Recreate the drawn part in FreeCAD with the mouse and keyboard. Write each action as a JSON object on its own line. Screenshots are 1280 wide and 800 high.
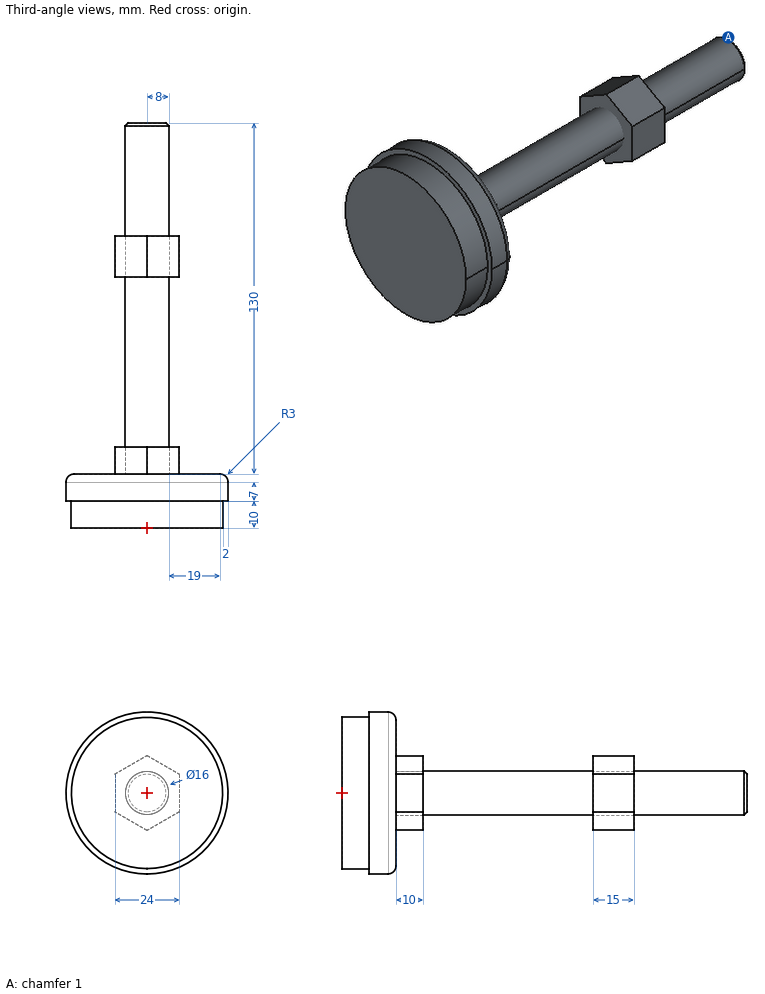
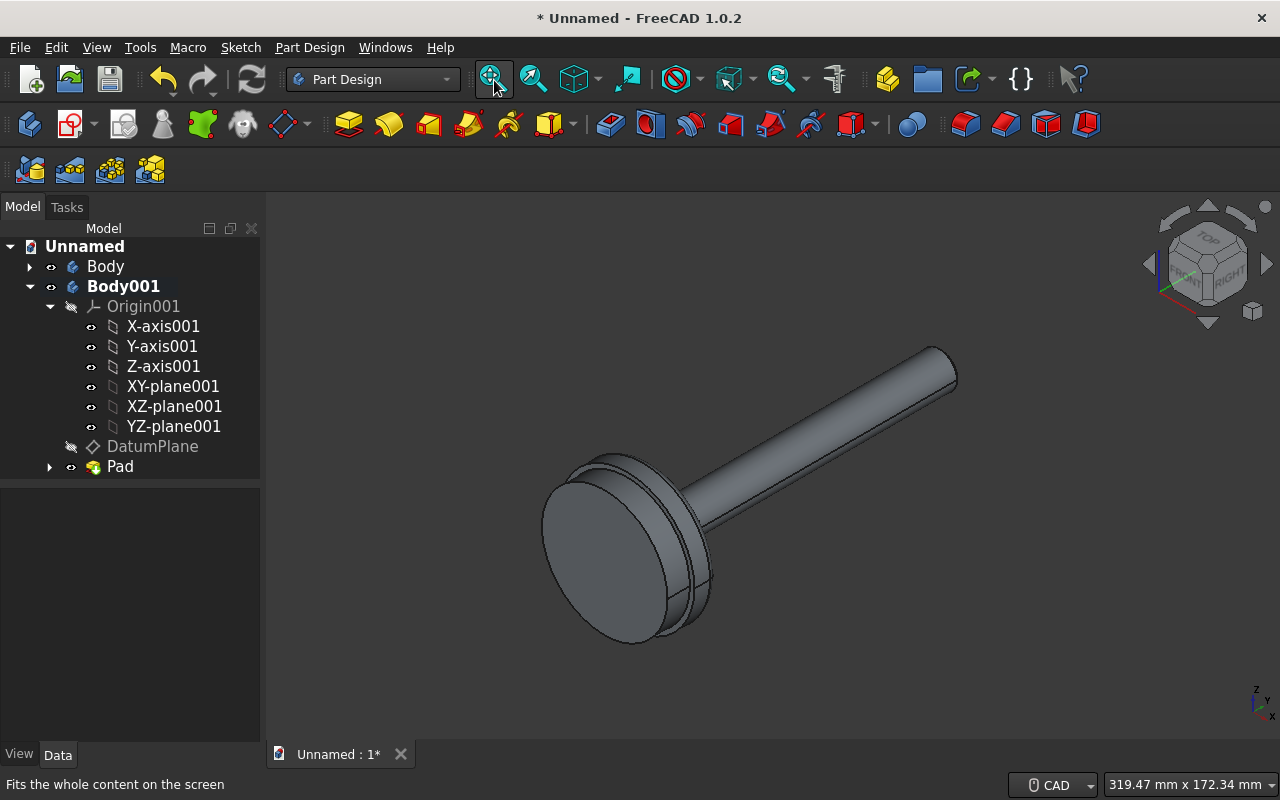
{"action": "left_click", "coordinate": [30, 124]}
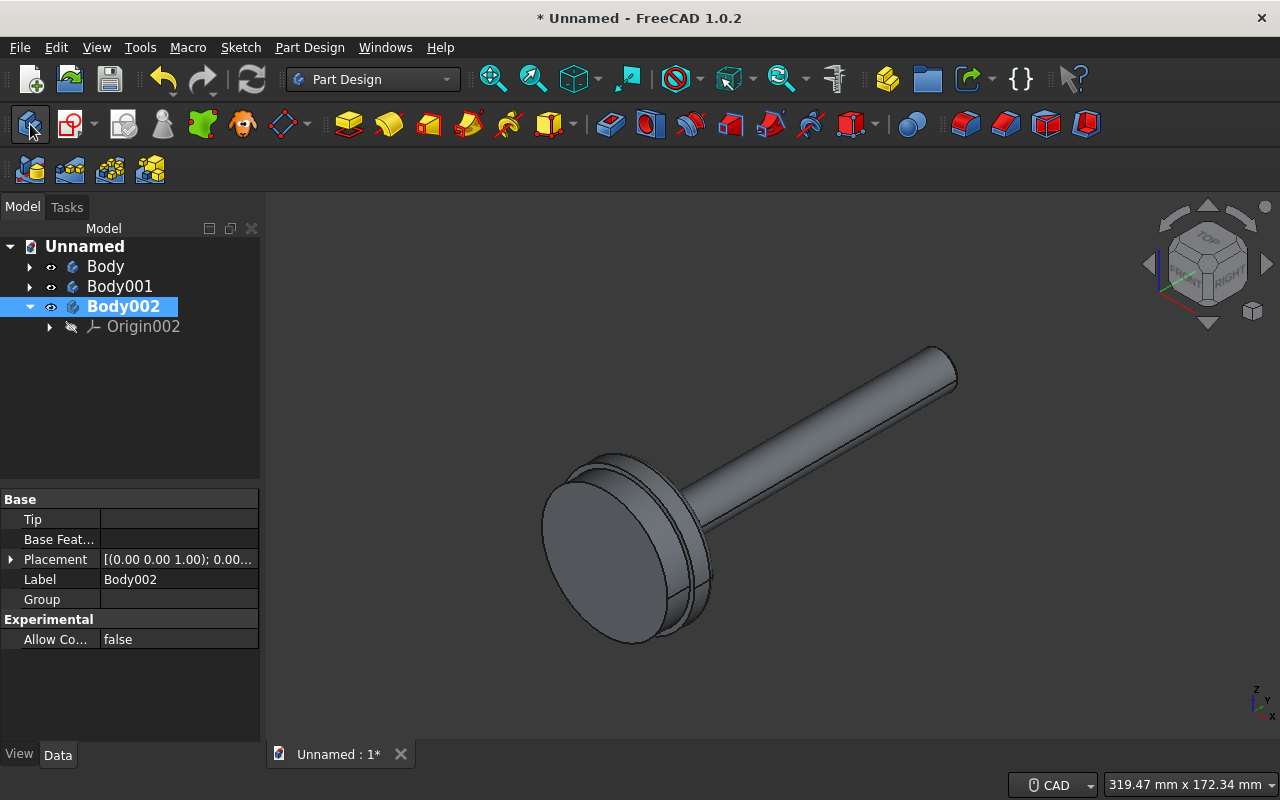
{"action": "left_click", "coordinate": [50, 327]}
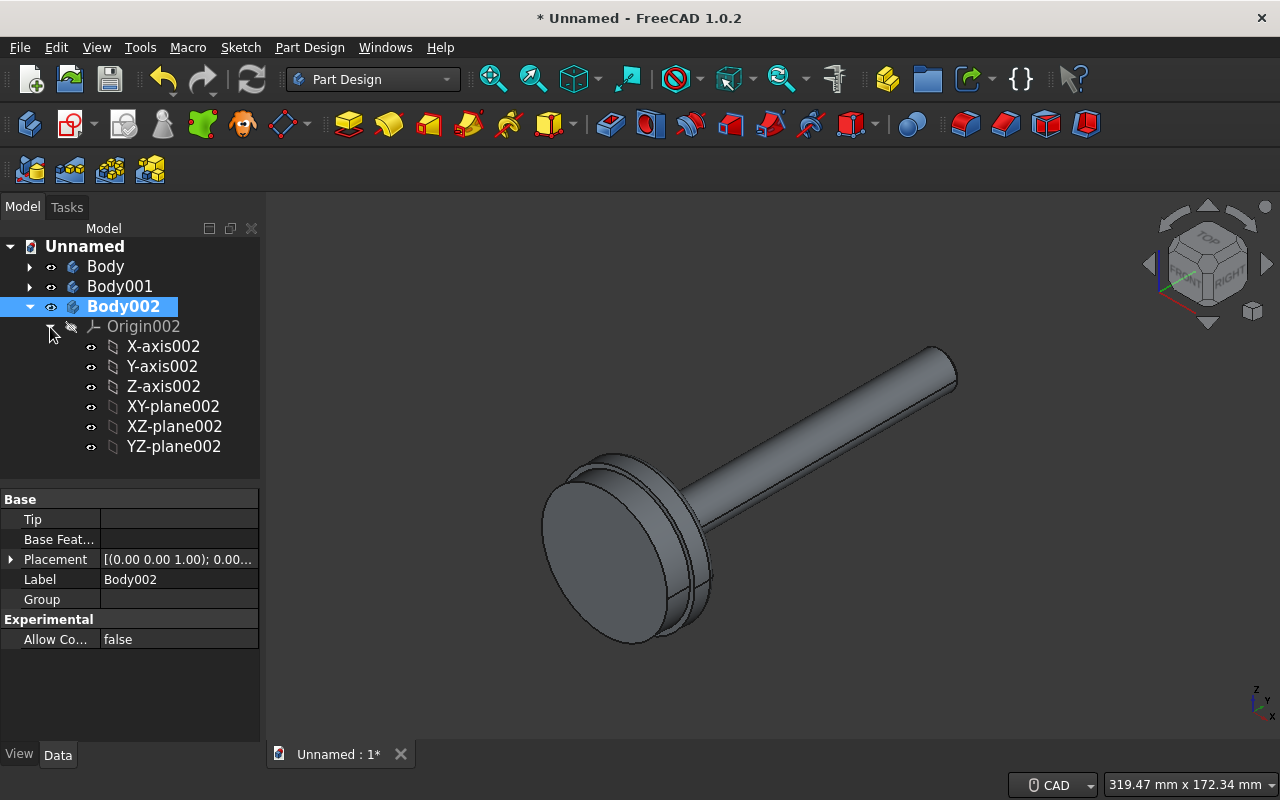
{"action": "left_click", "coordinate": [136, 427]}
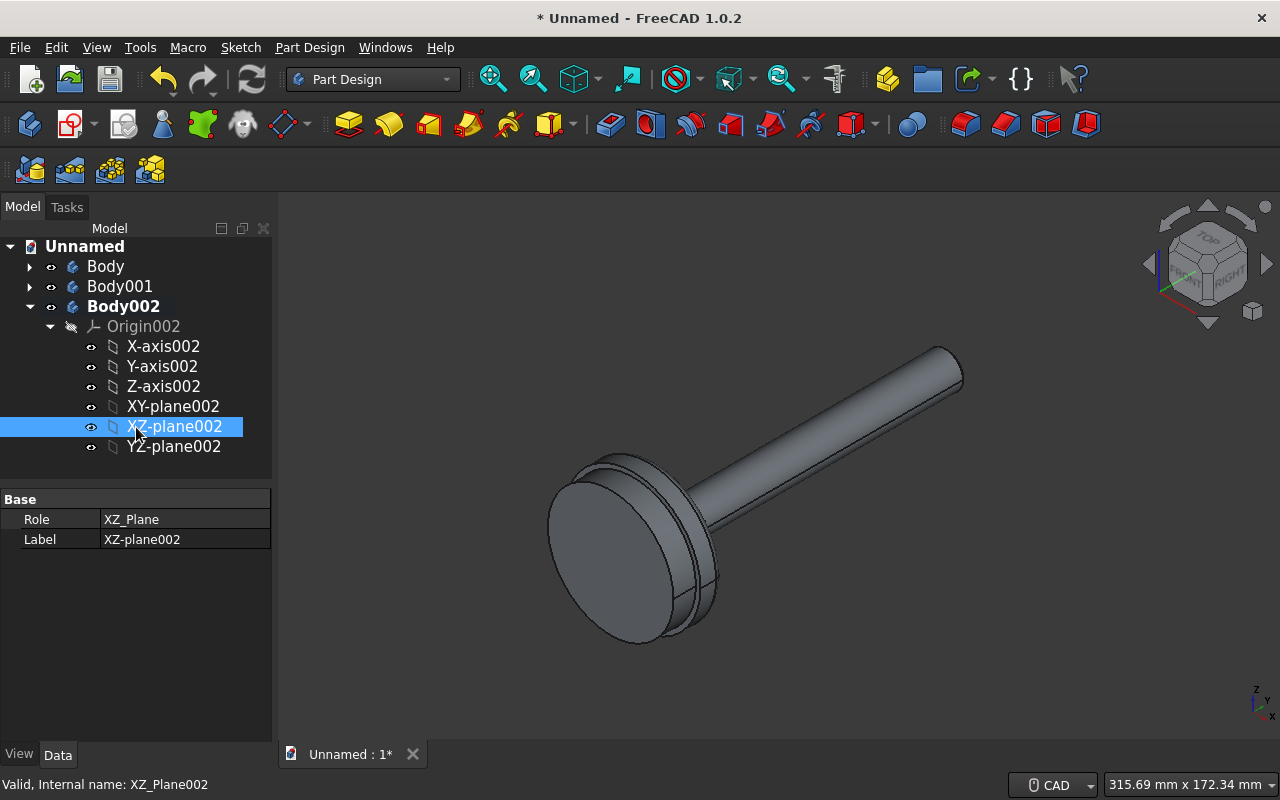
{"action": "left_click", "coordinate": [284, 124]}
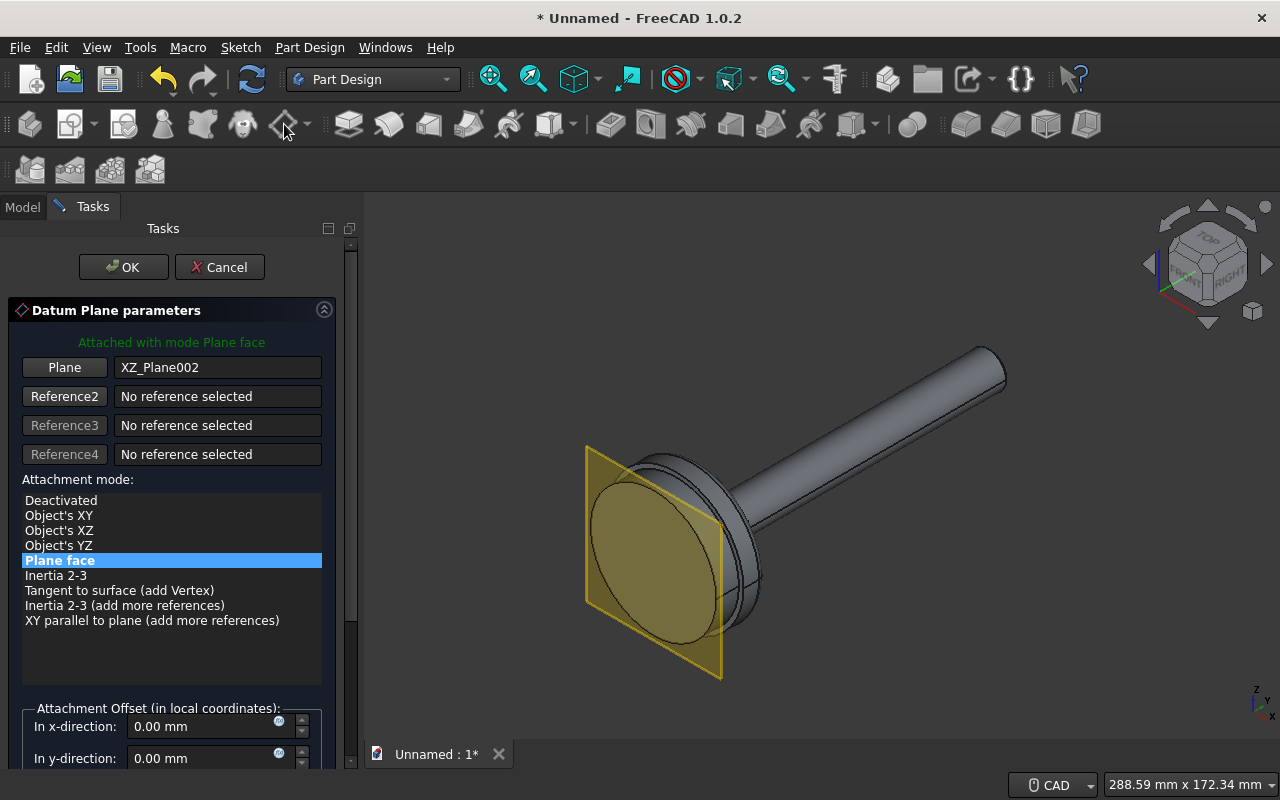
{"action": "scroll", "coordinate": [351, 503], "scroll_direction": "down", "scroll_amount": 2}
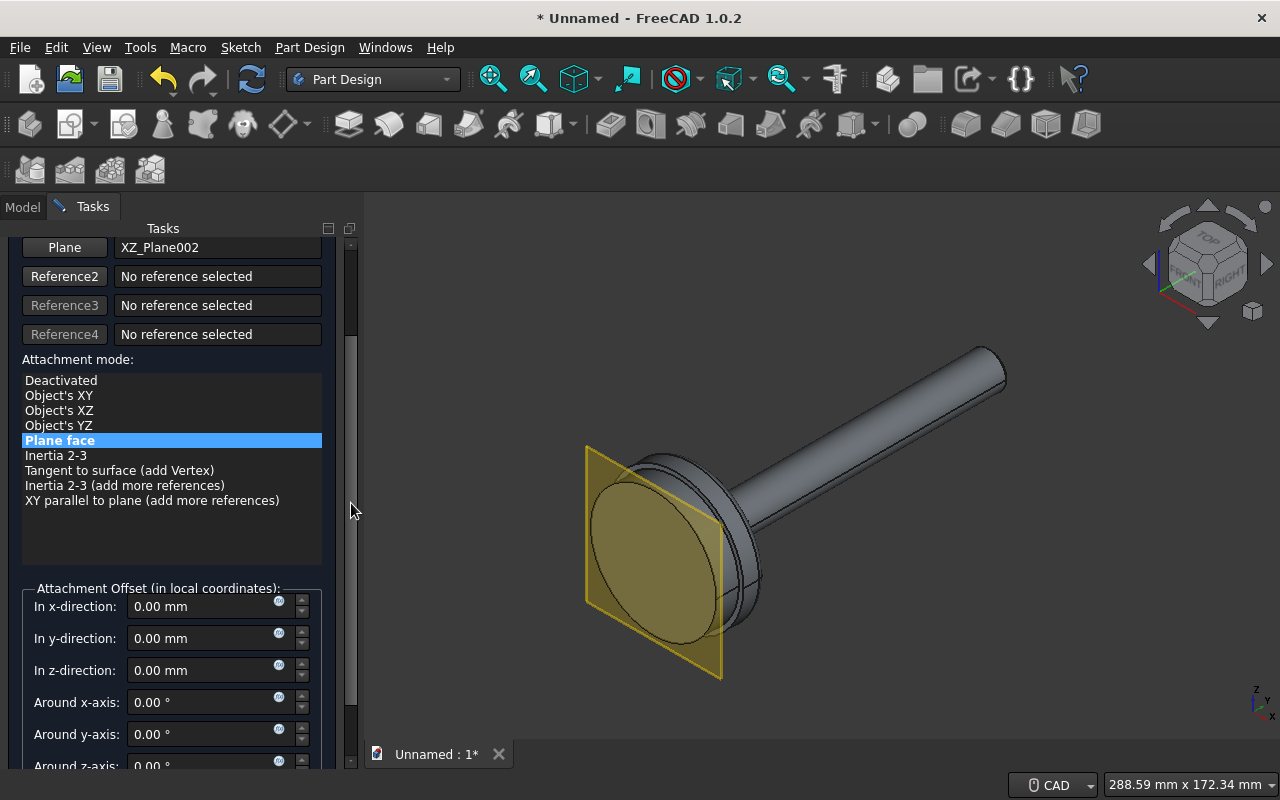
{"action": "triple_click", "coordinate": [210, 670]}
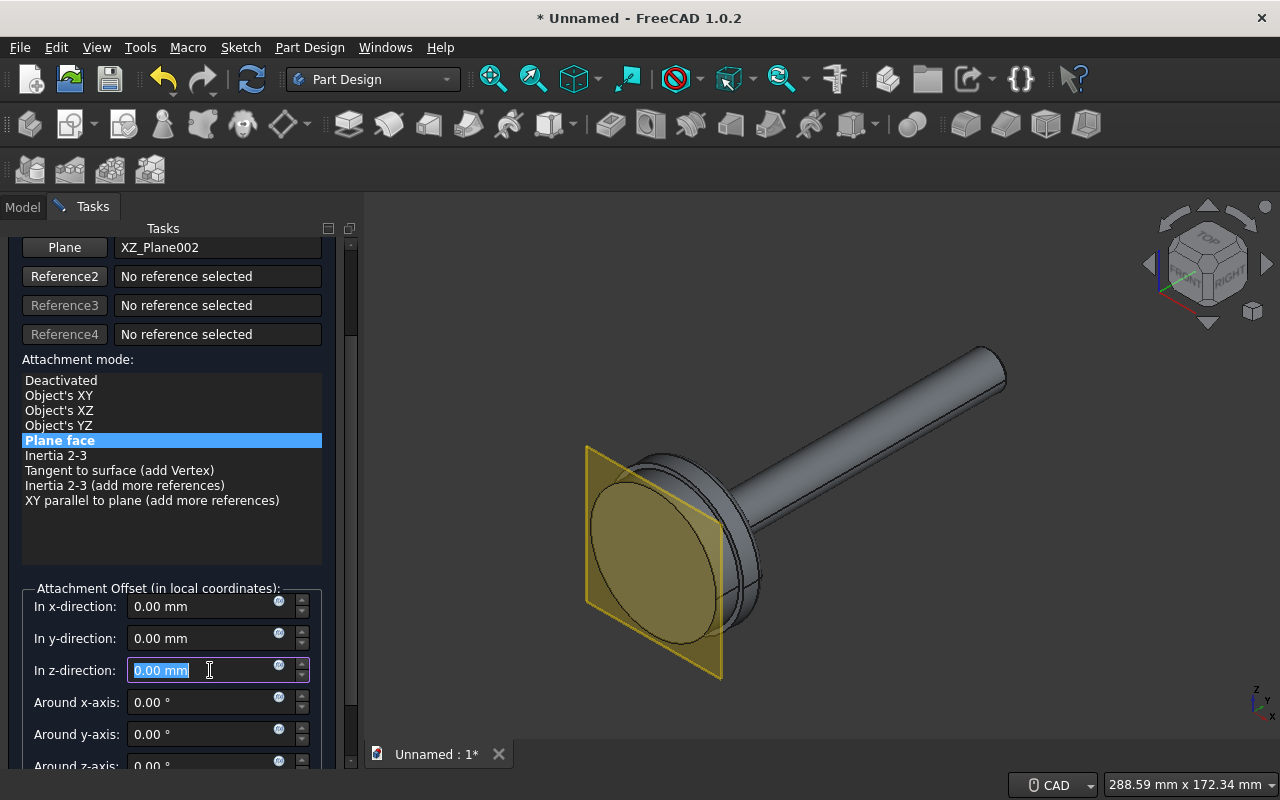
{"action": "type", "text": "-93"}
{"action": "key", "text": "Tab"}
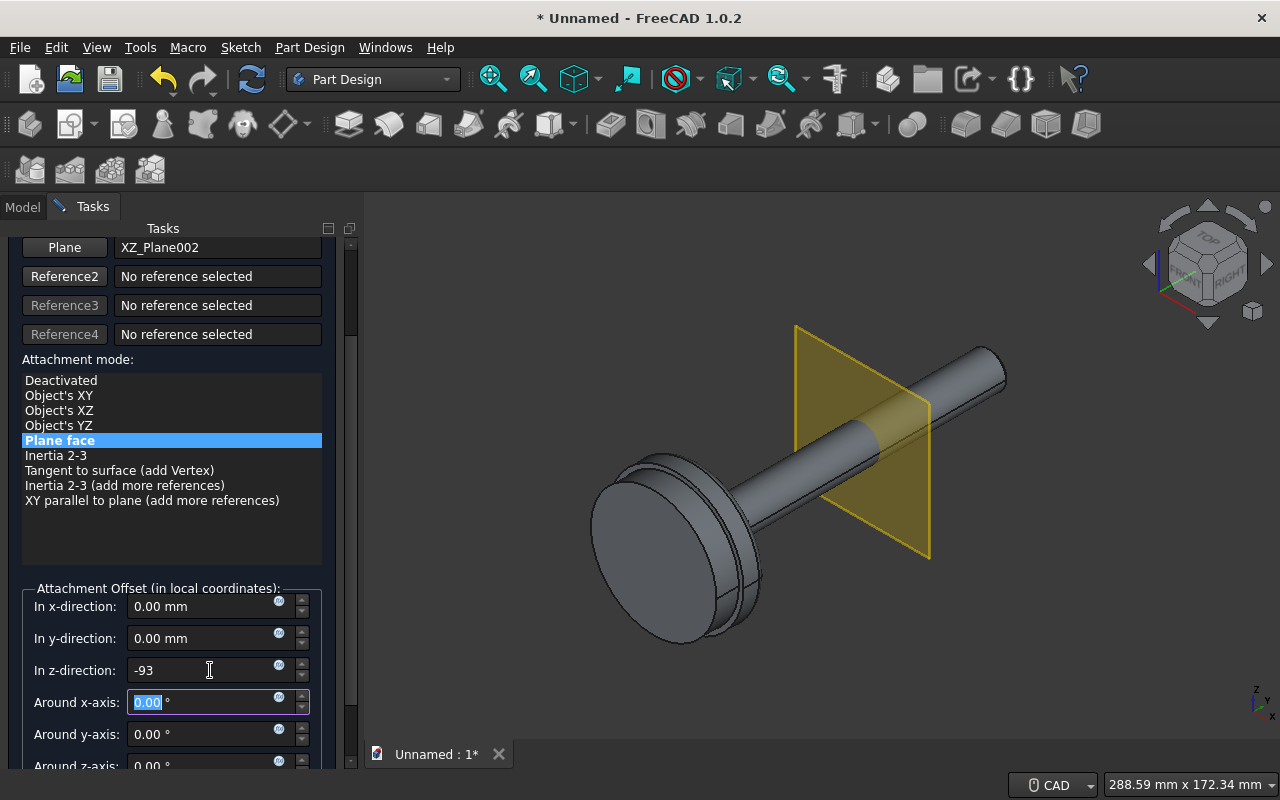
{"action": "scroll", "coordinate": [351, 503], "scroll_direction": "up", "scroll_amount": 3}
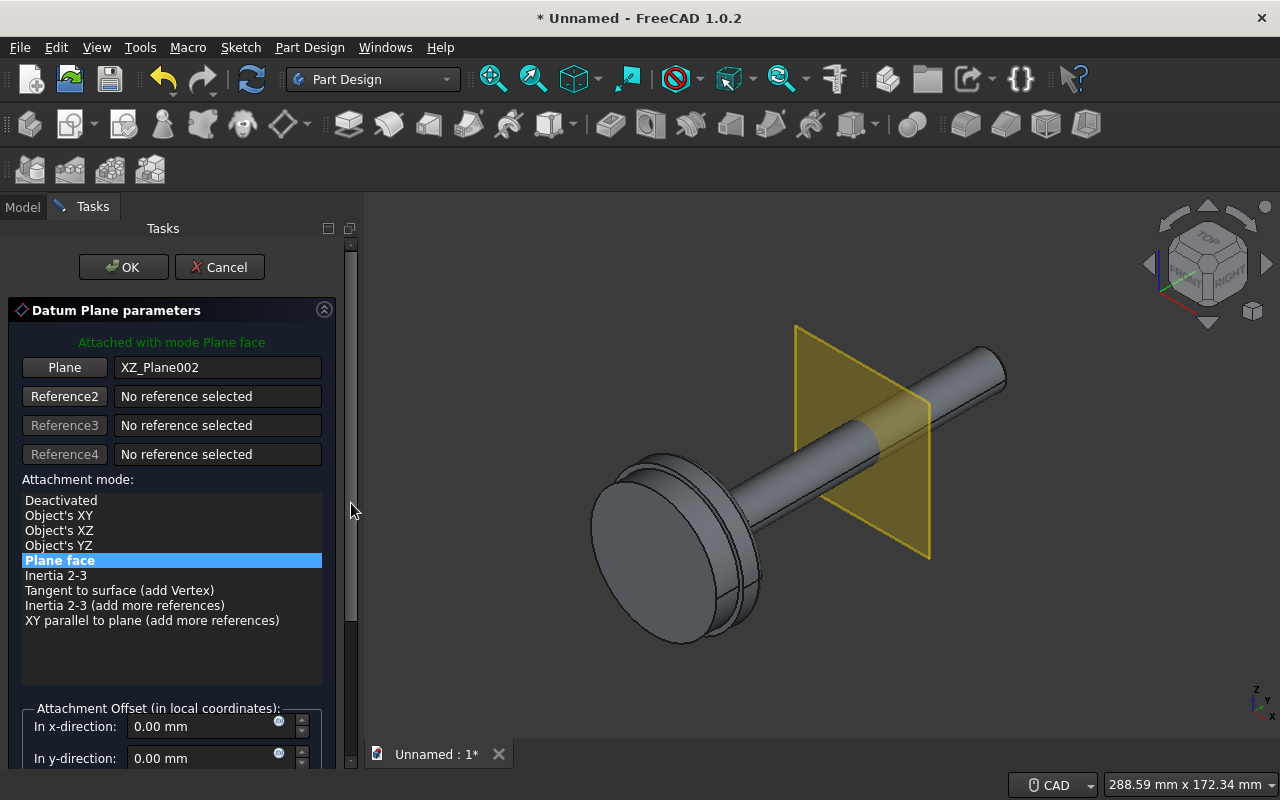
{"action": "left_click", "coordinate": [124, 267]}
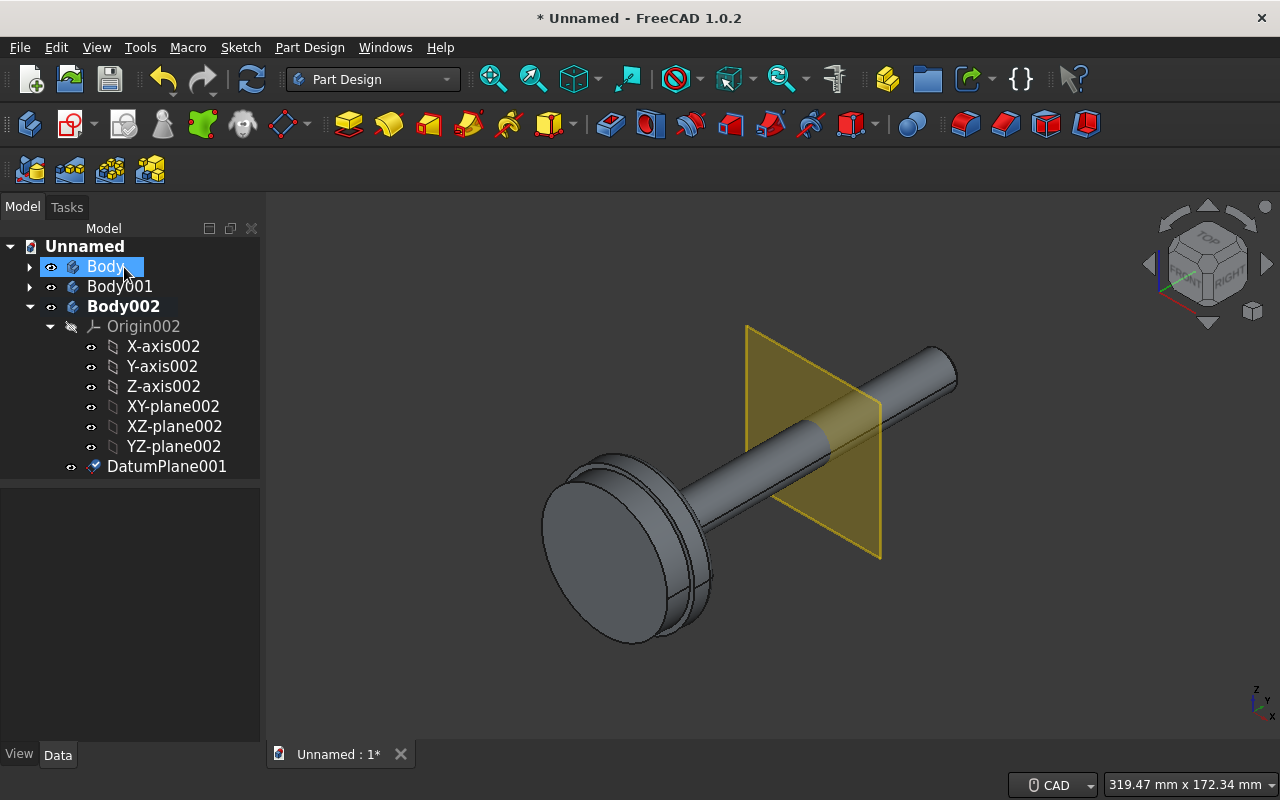
{"action": "left_click", "coordinate": [116, 467]}